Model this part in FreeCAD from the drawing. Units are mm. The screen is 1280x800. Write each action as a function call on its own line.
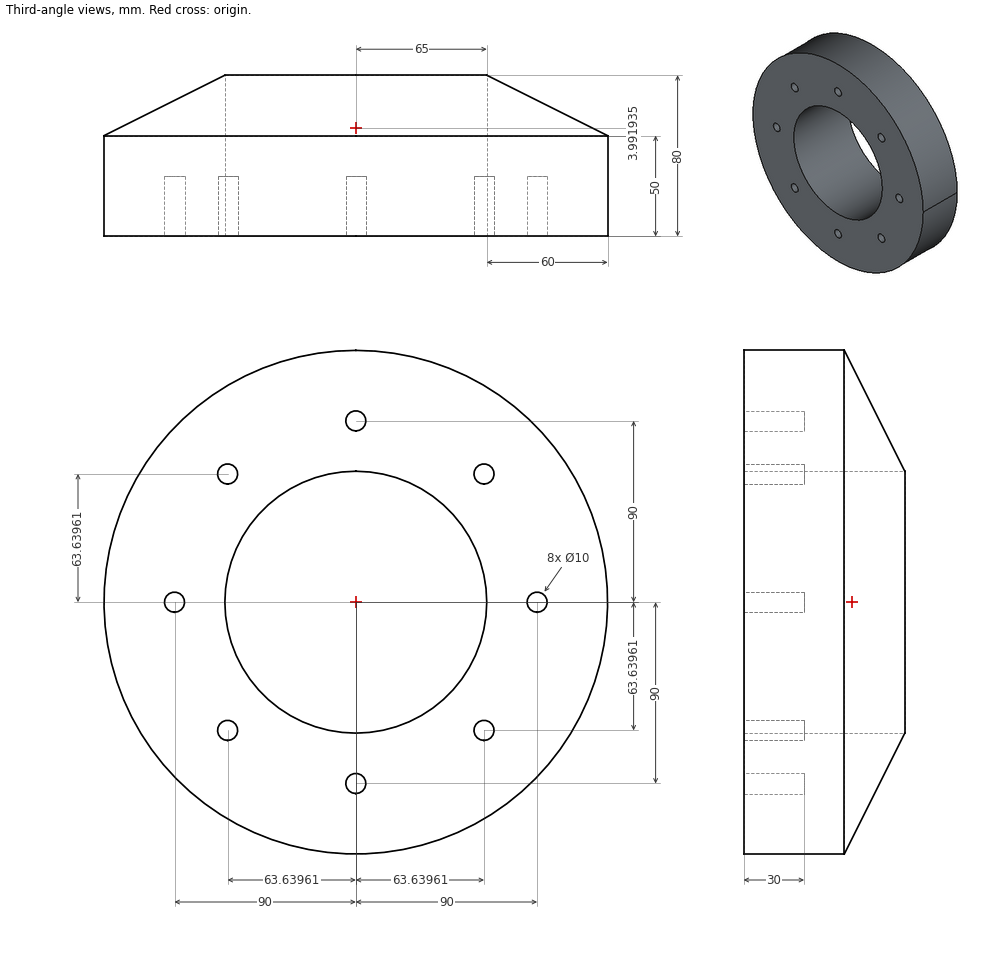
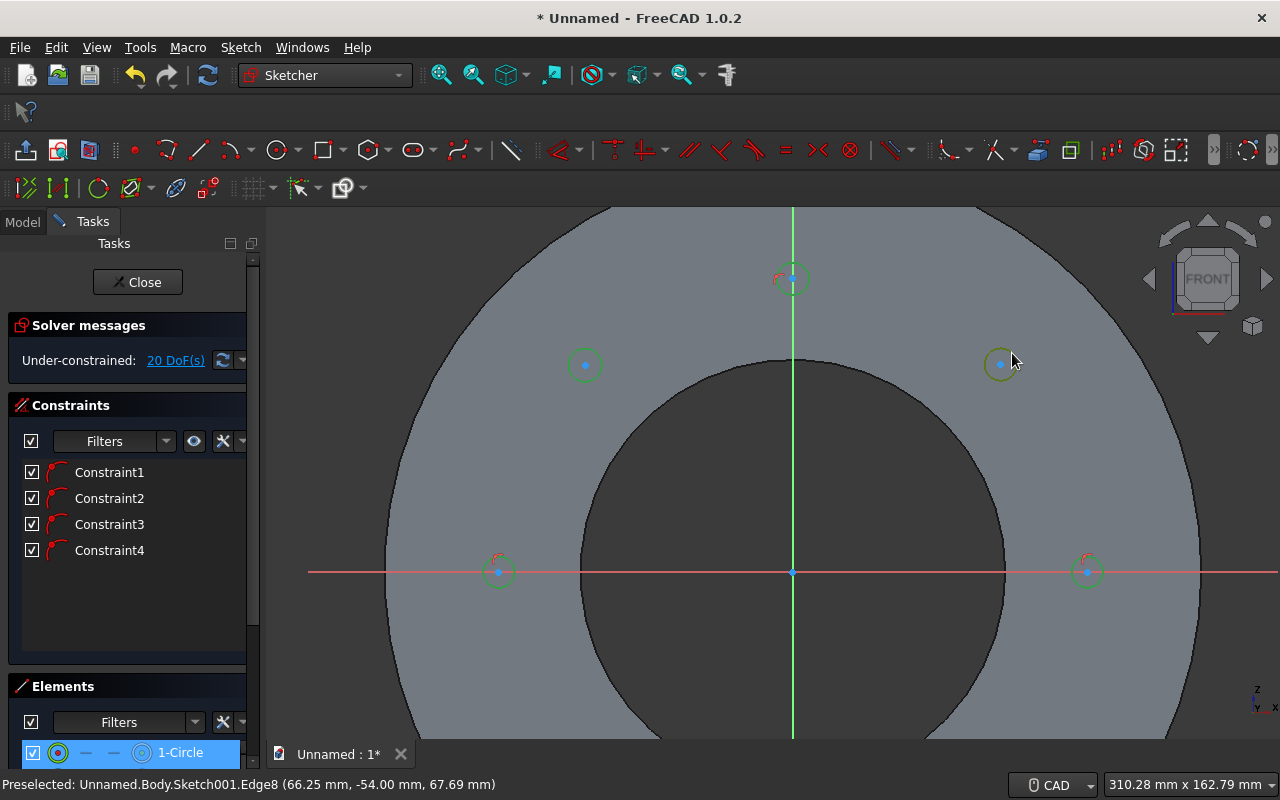
click(786, 150)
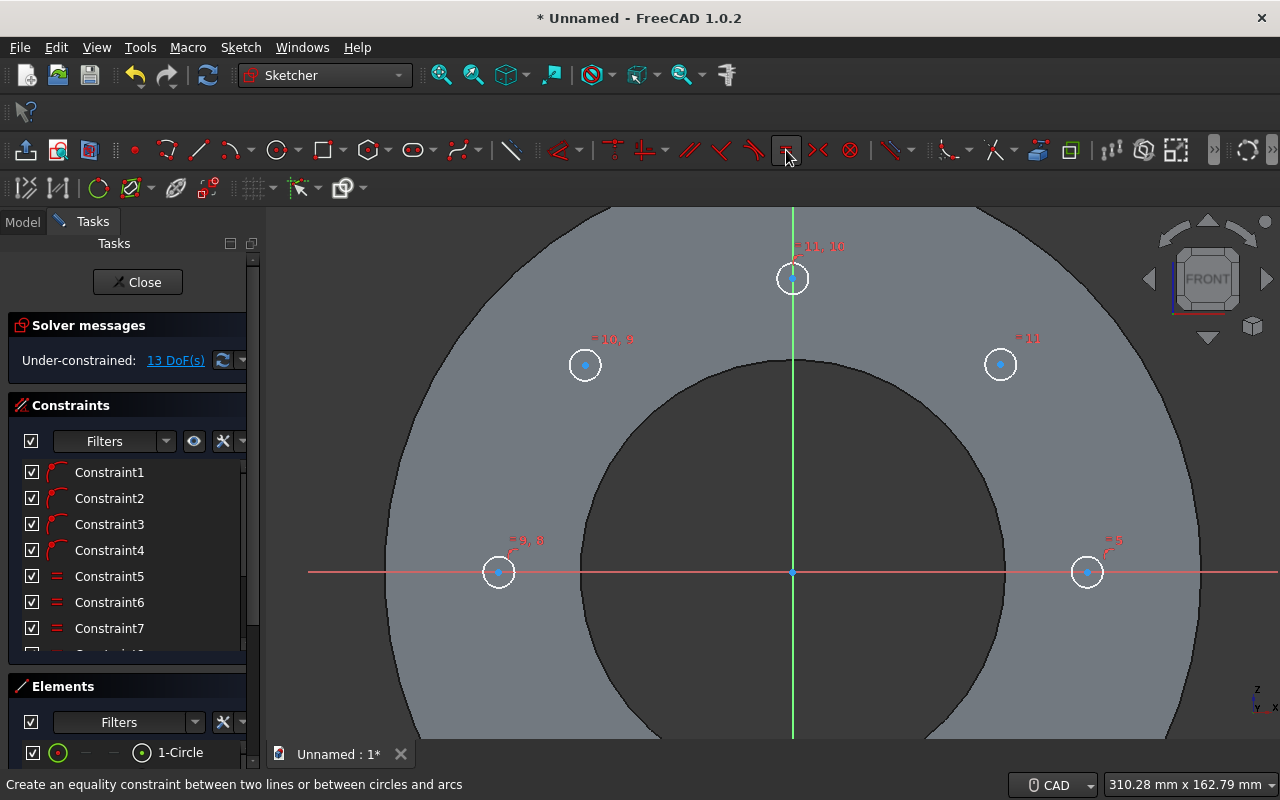
scroll(597, 352, down, 3)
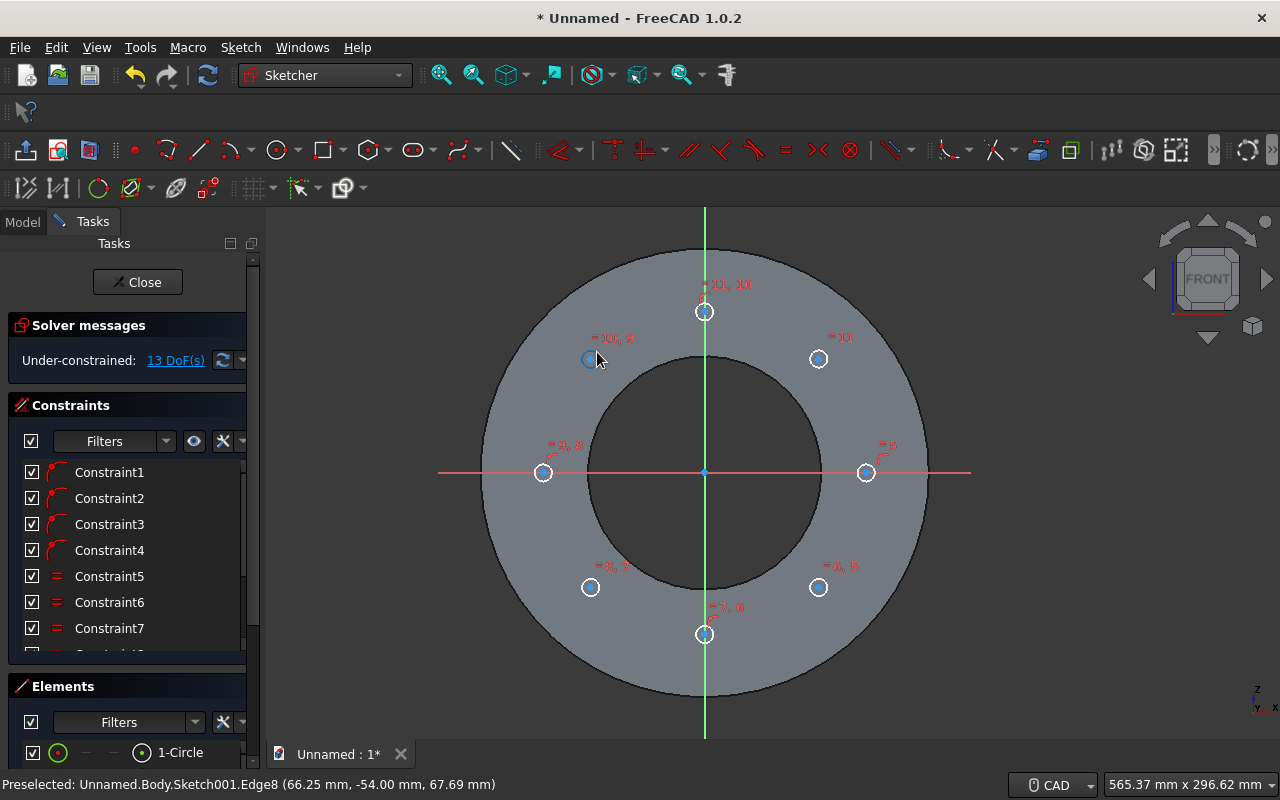
click(819, 588)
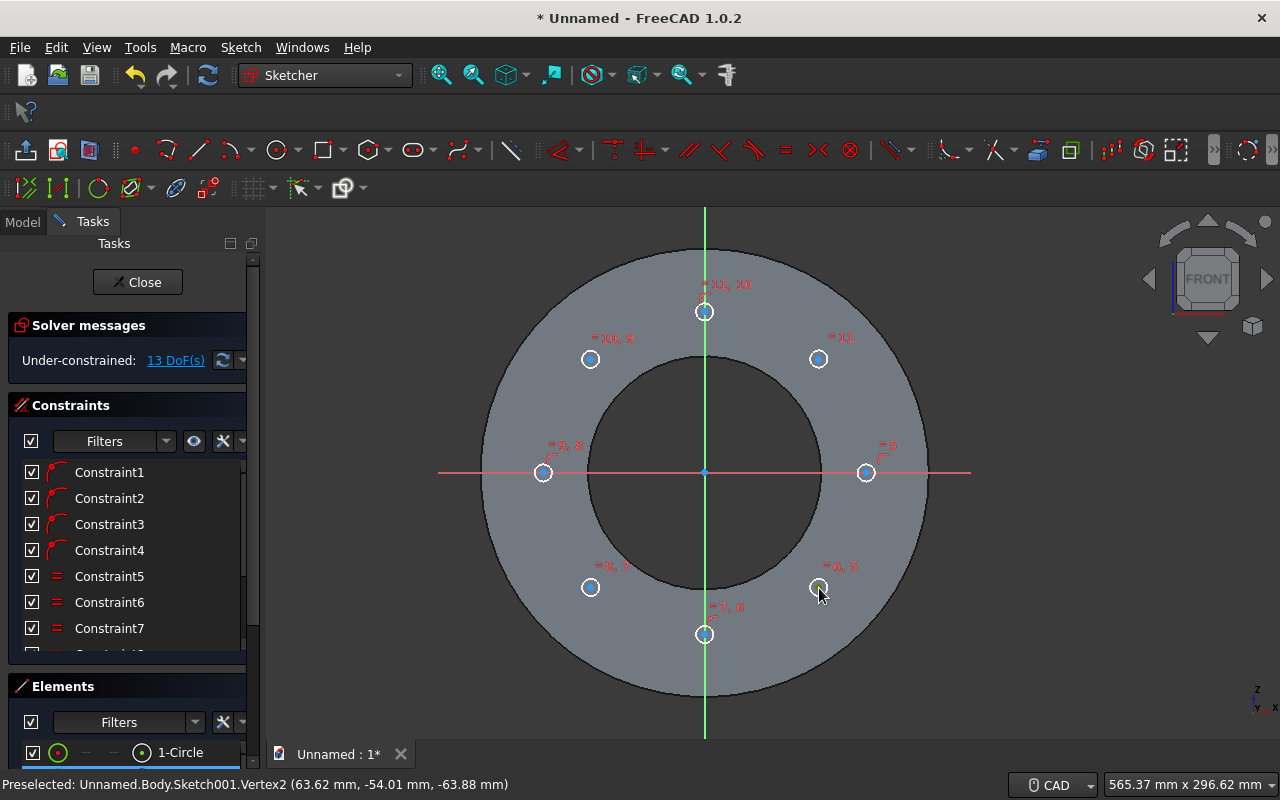
click(591, 587)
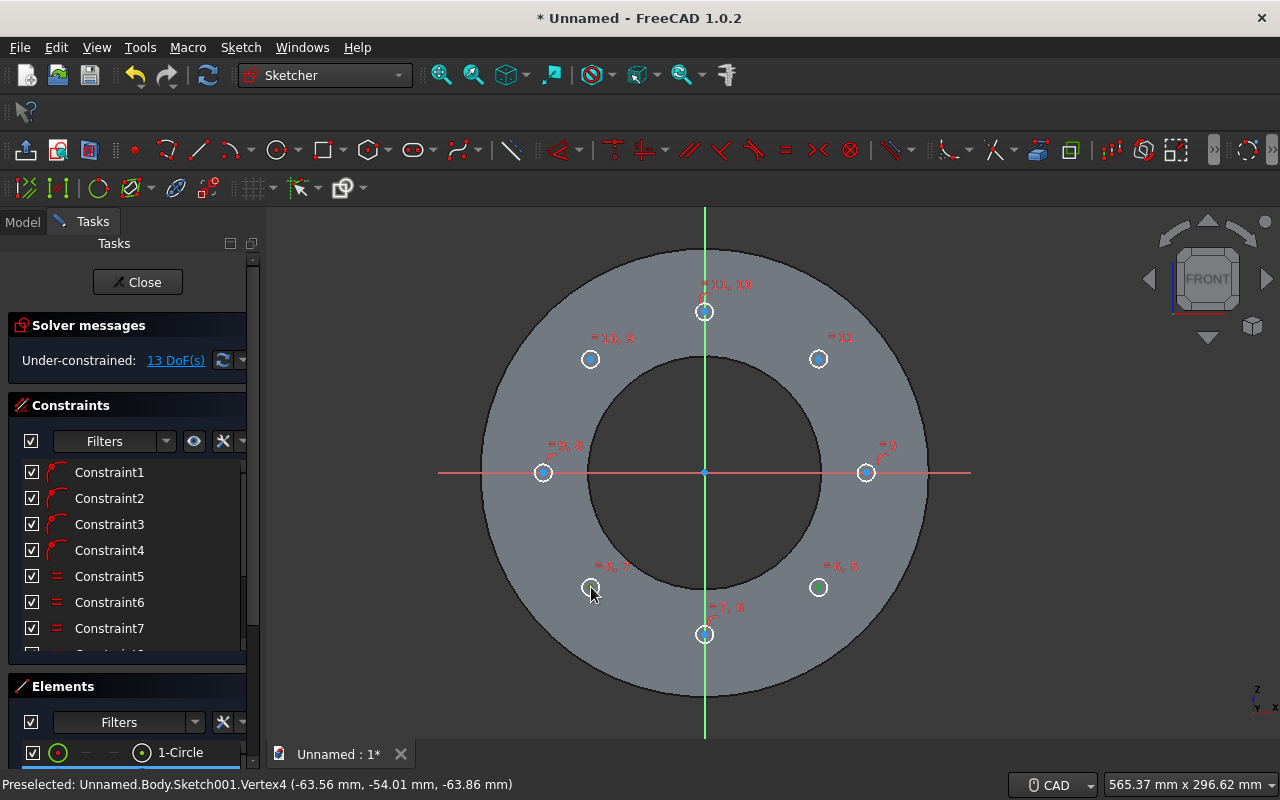
key(h)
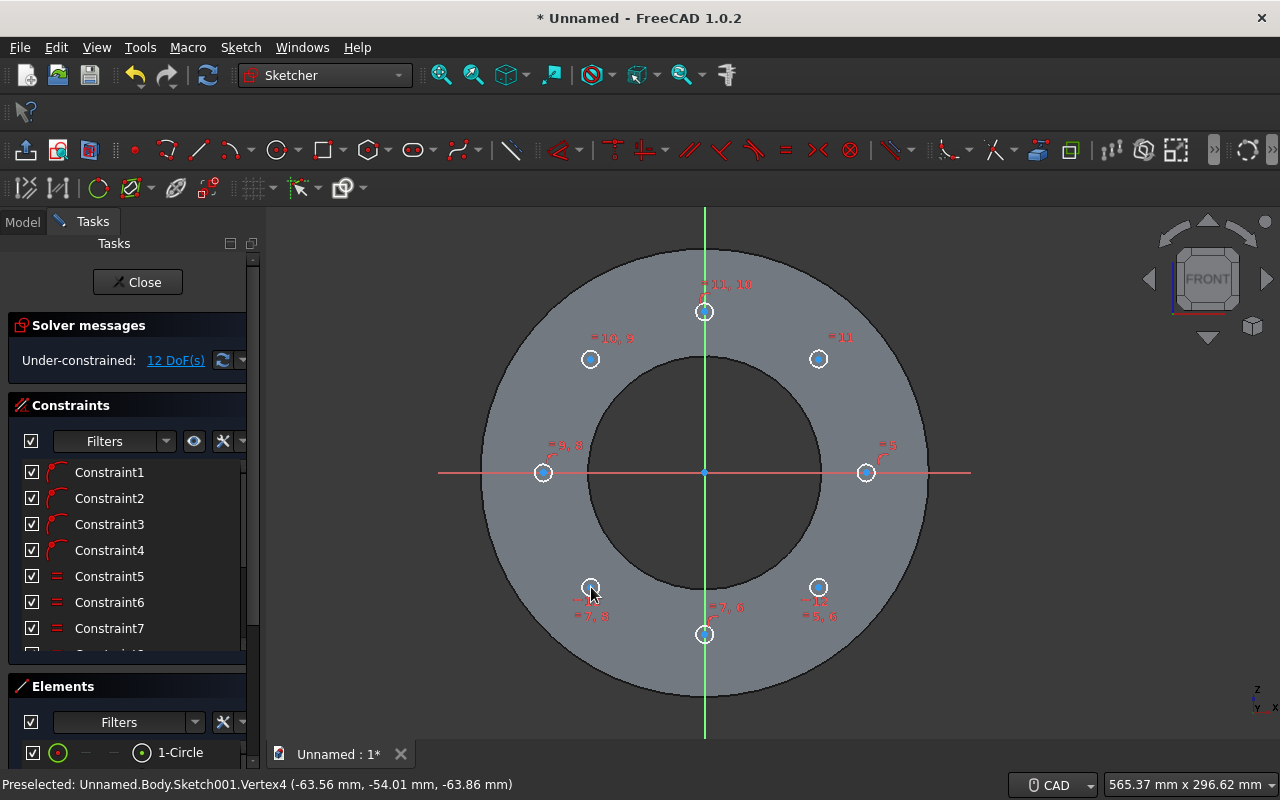
click(591, 588)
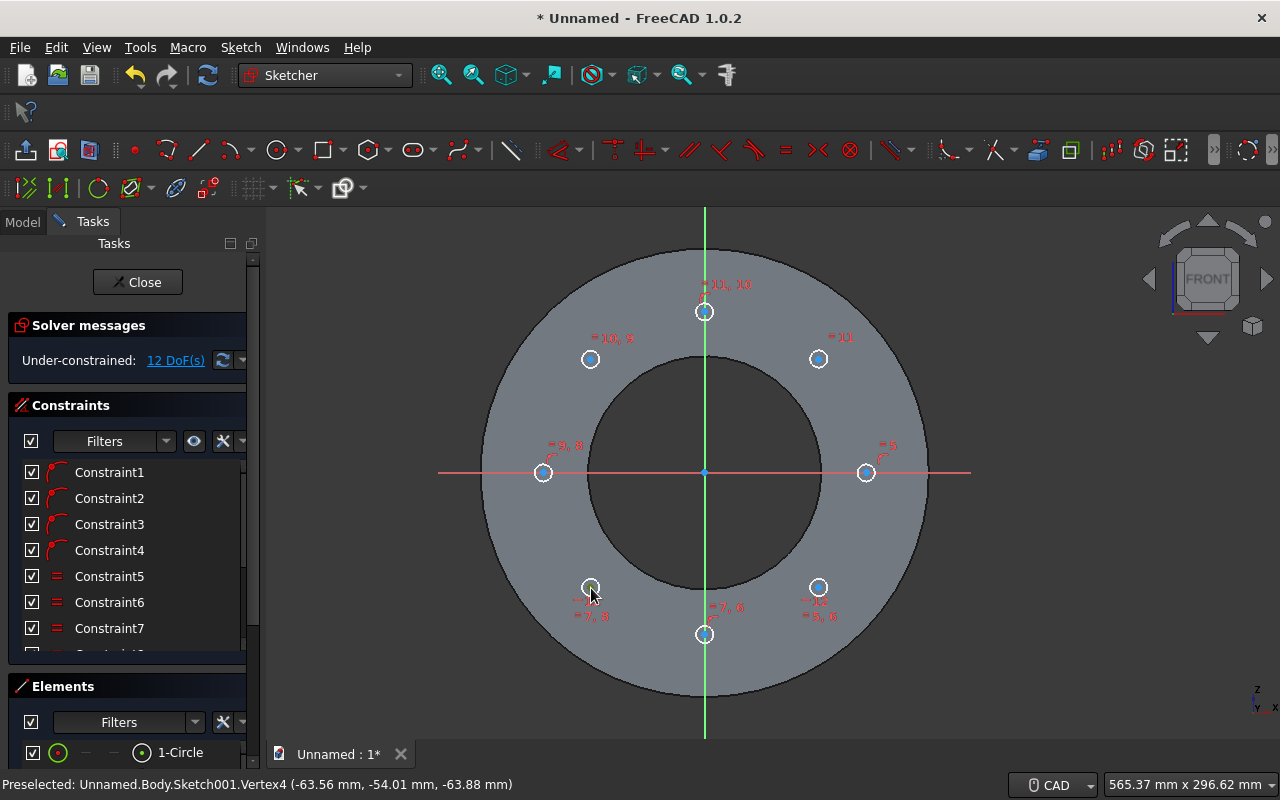
click(591, 359)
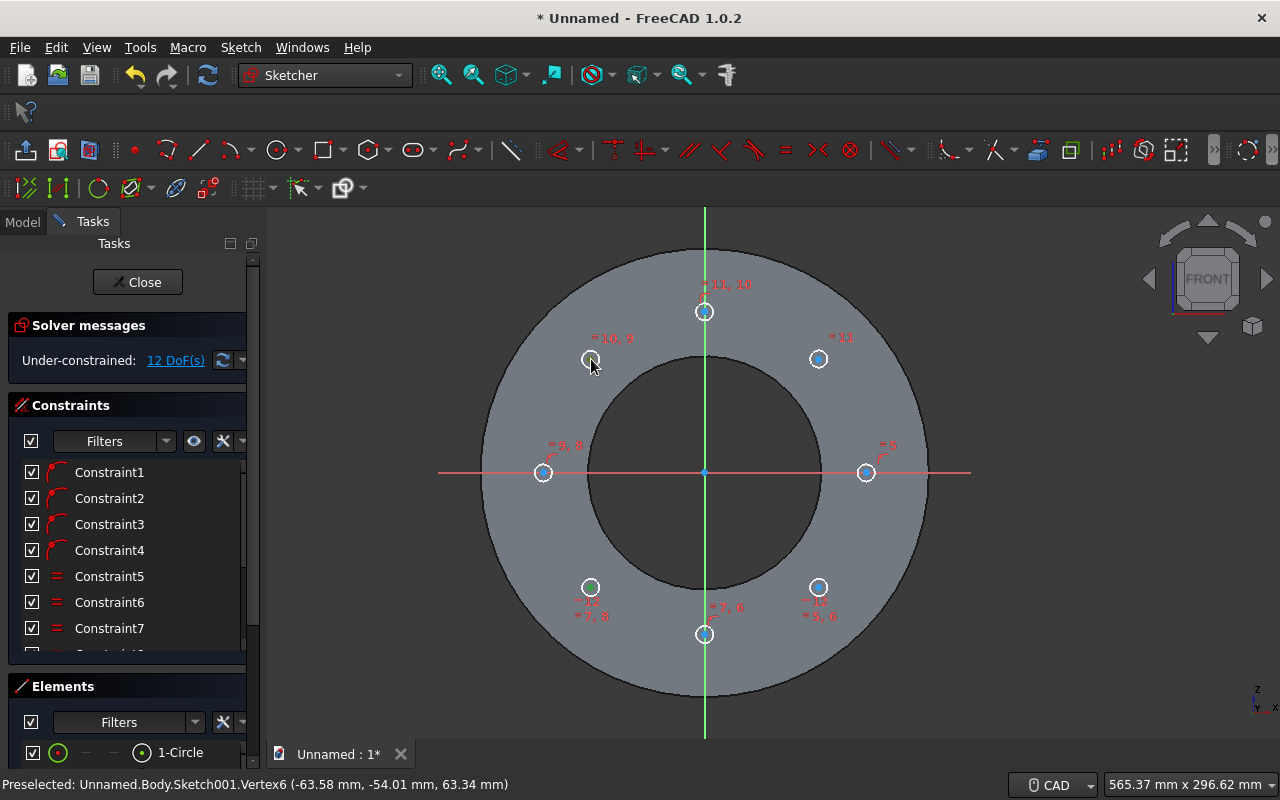
click(668, 150)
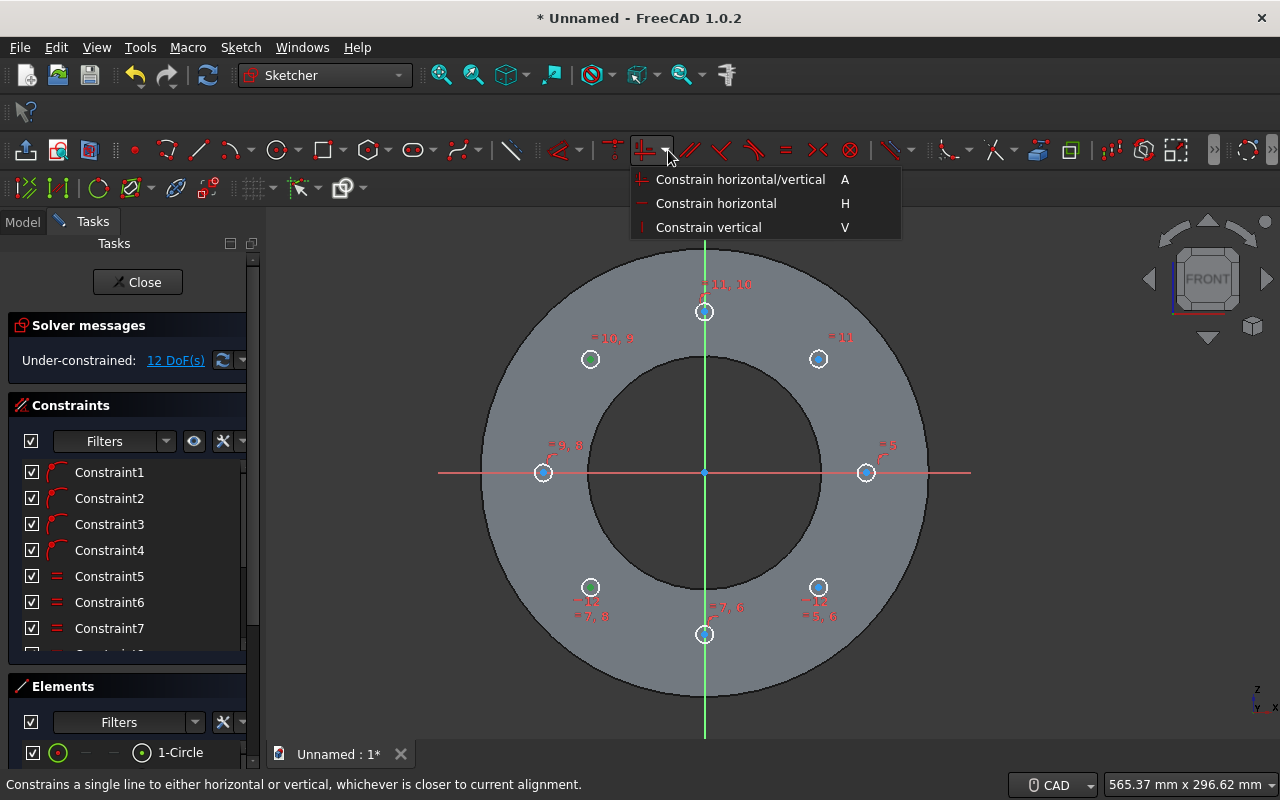
click(766, 227)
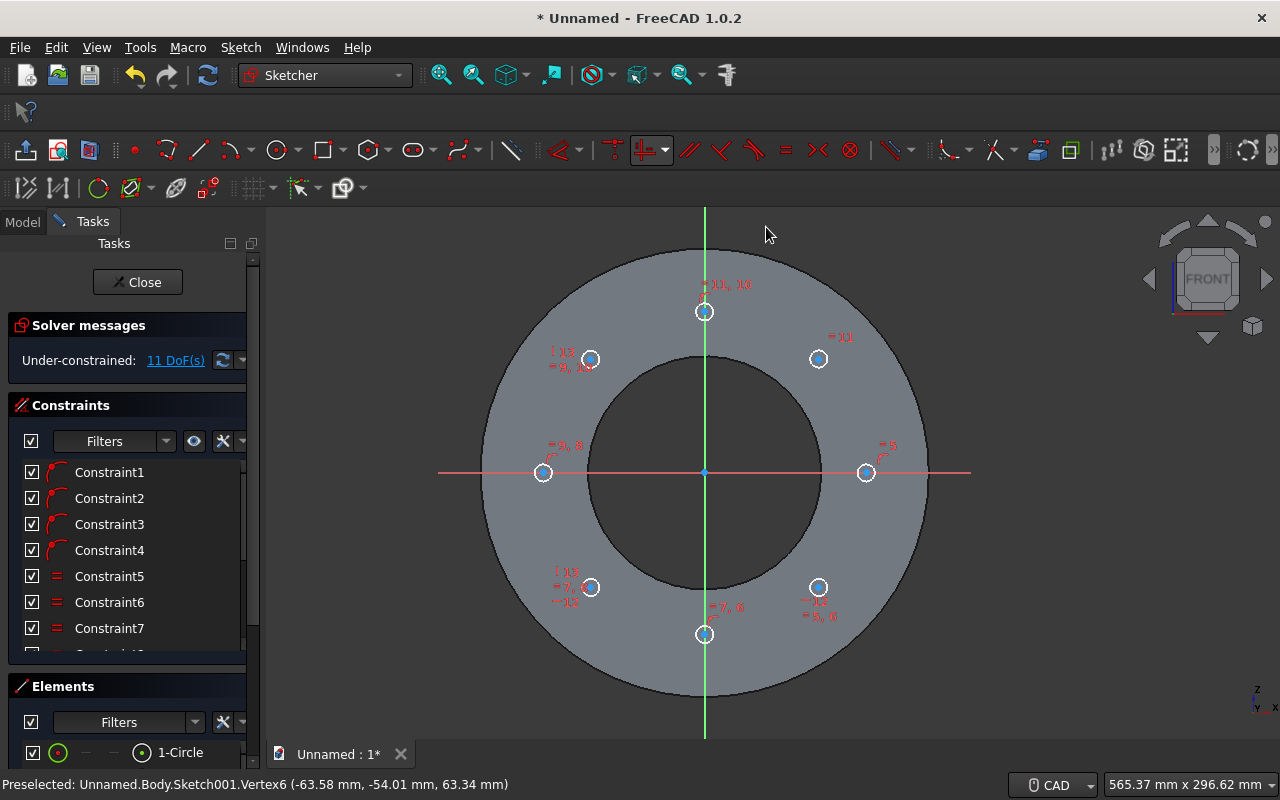
click(819, 588)